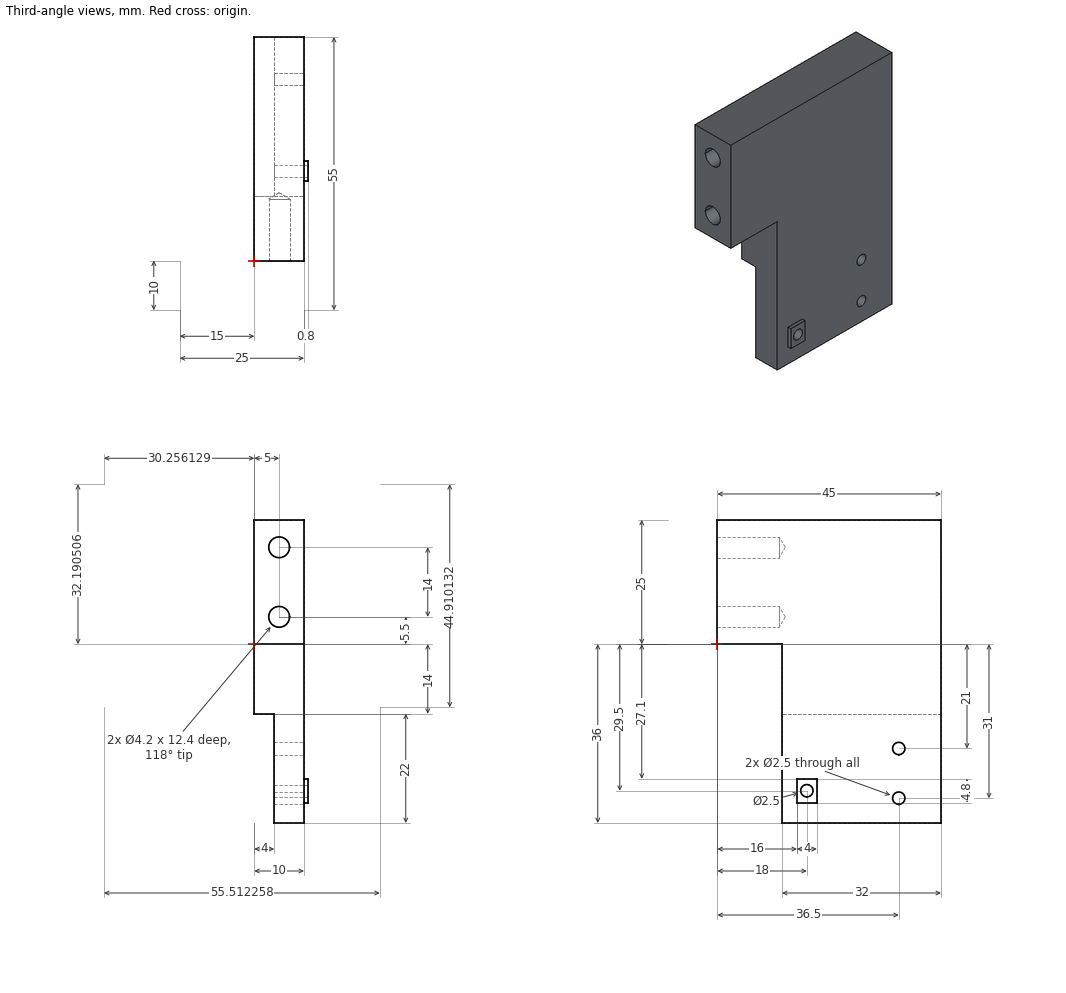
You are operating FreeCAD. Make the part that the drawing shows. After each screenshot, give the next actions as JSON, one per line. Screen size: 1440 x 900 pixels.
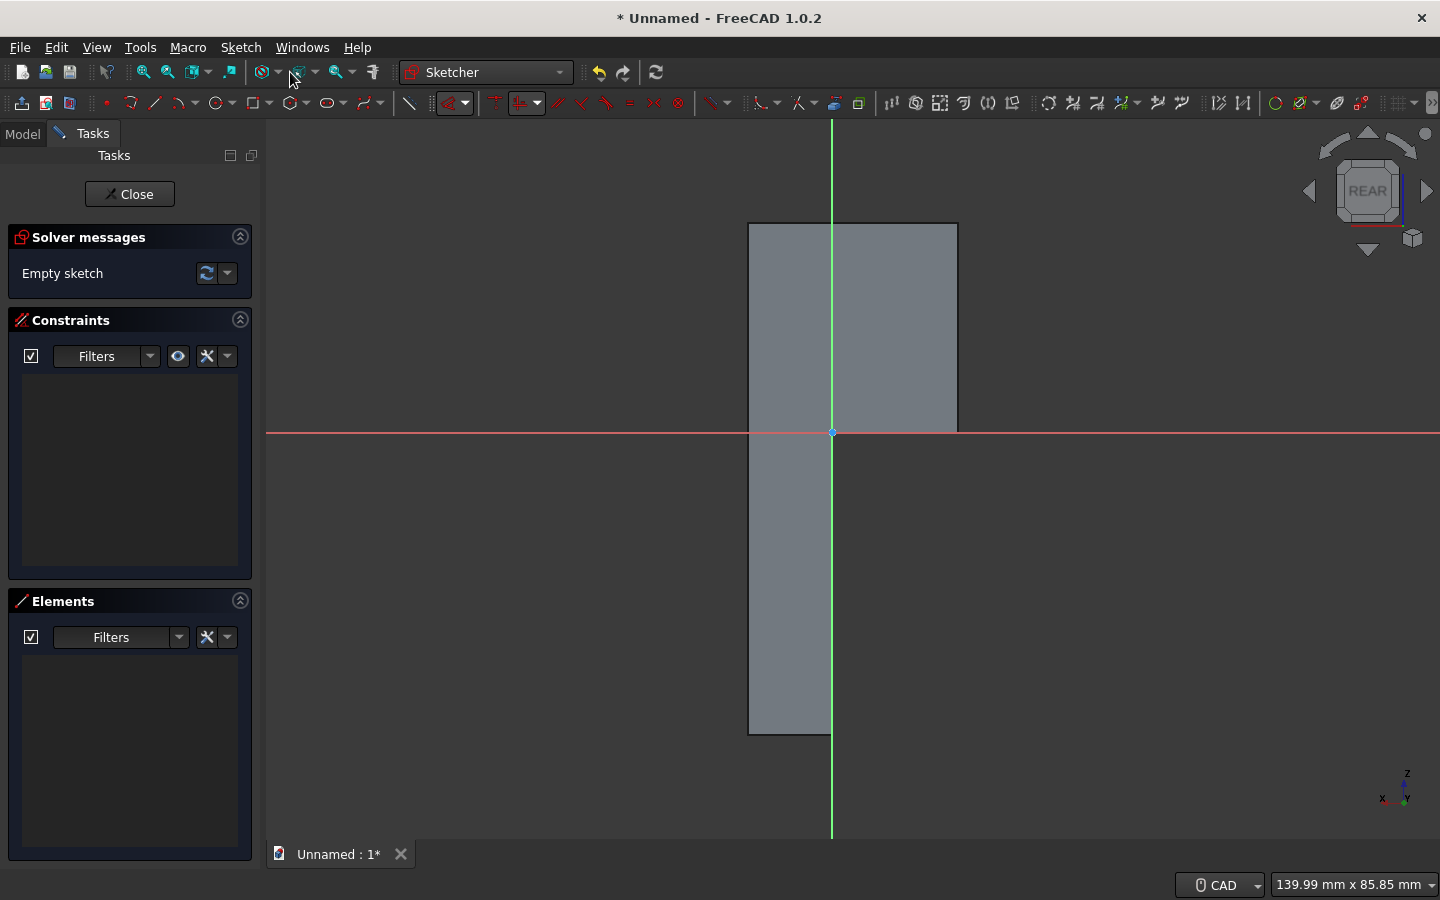
{"action": "scroll", "coordinate": [878, 797], "scroll_direction": "up", "scroll_amount": 2}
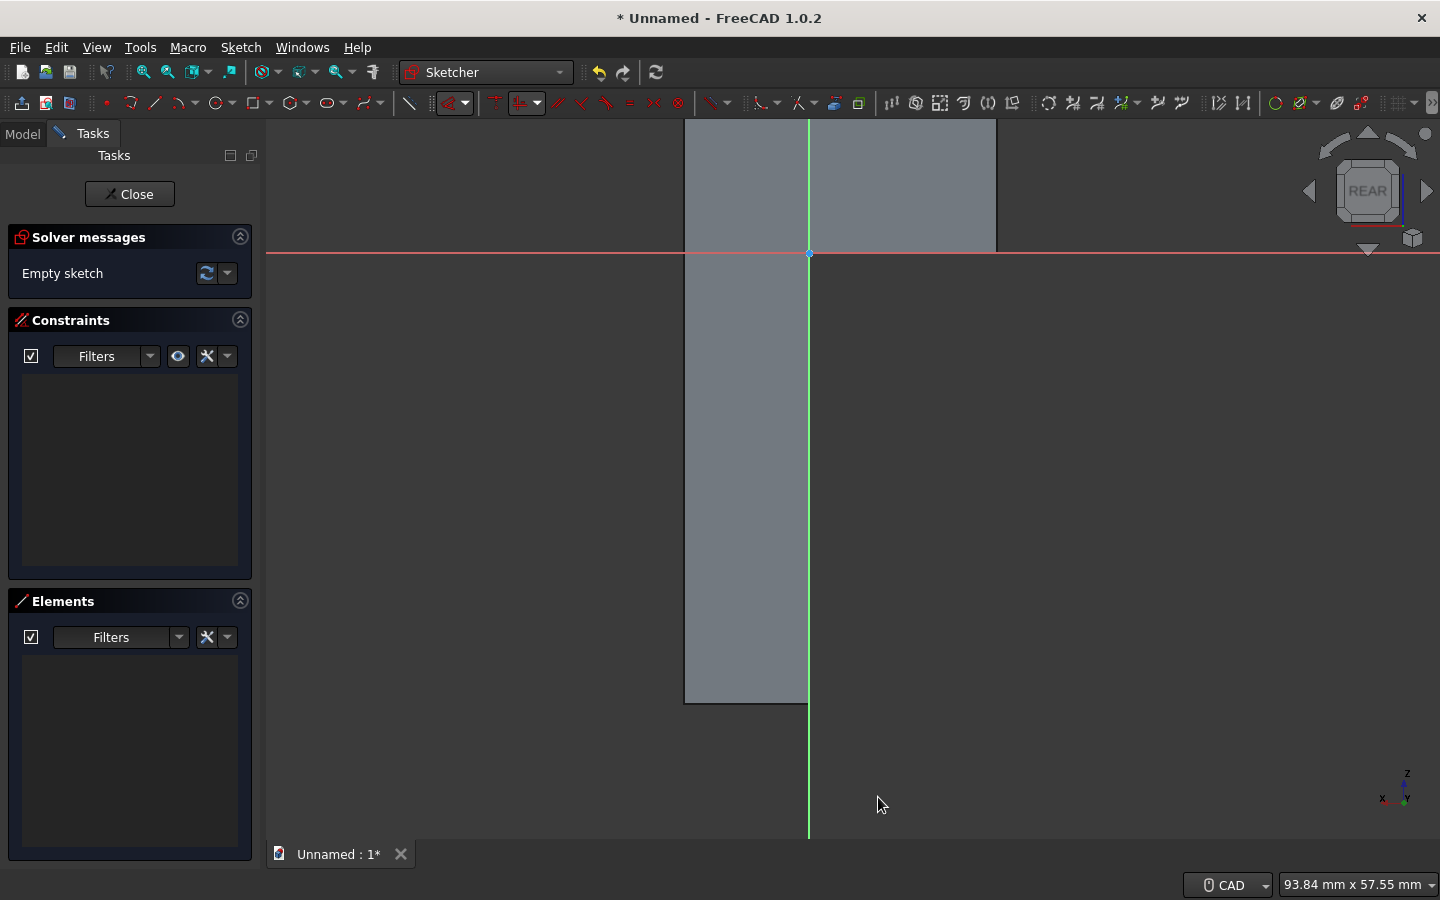
{"action": "key", "text": "g r"}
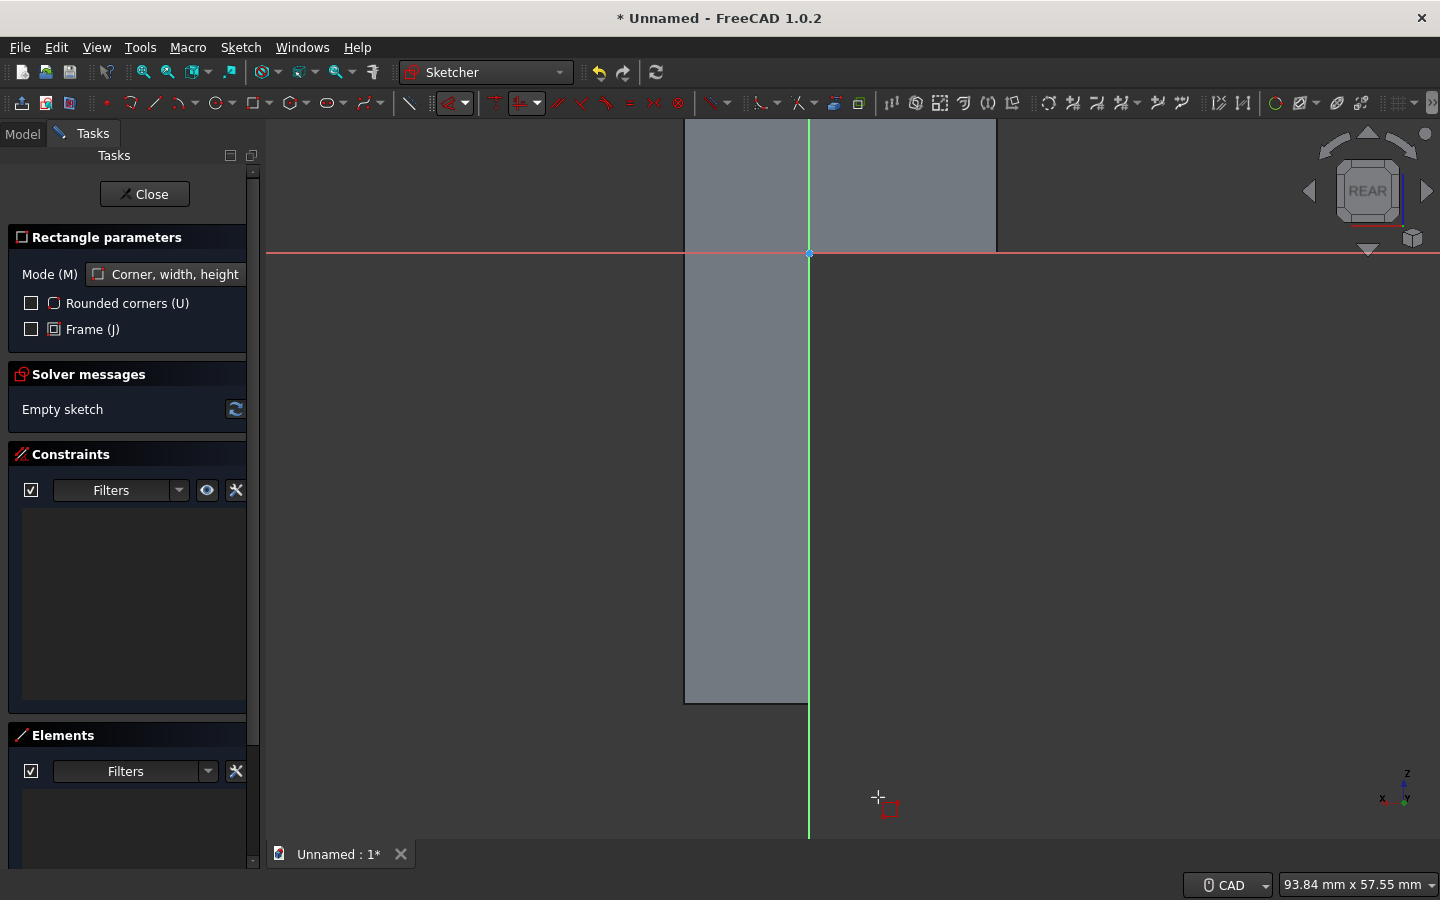
{"action": "left_click", "coordinate": [759, 428]}
{"action": "left_click", "coordinate": [809, 704]}
{"action": "key", "text": "Escape"}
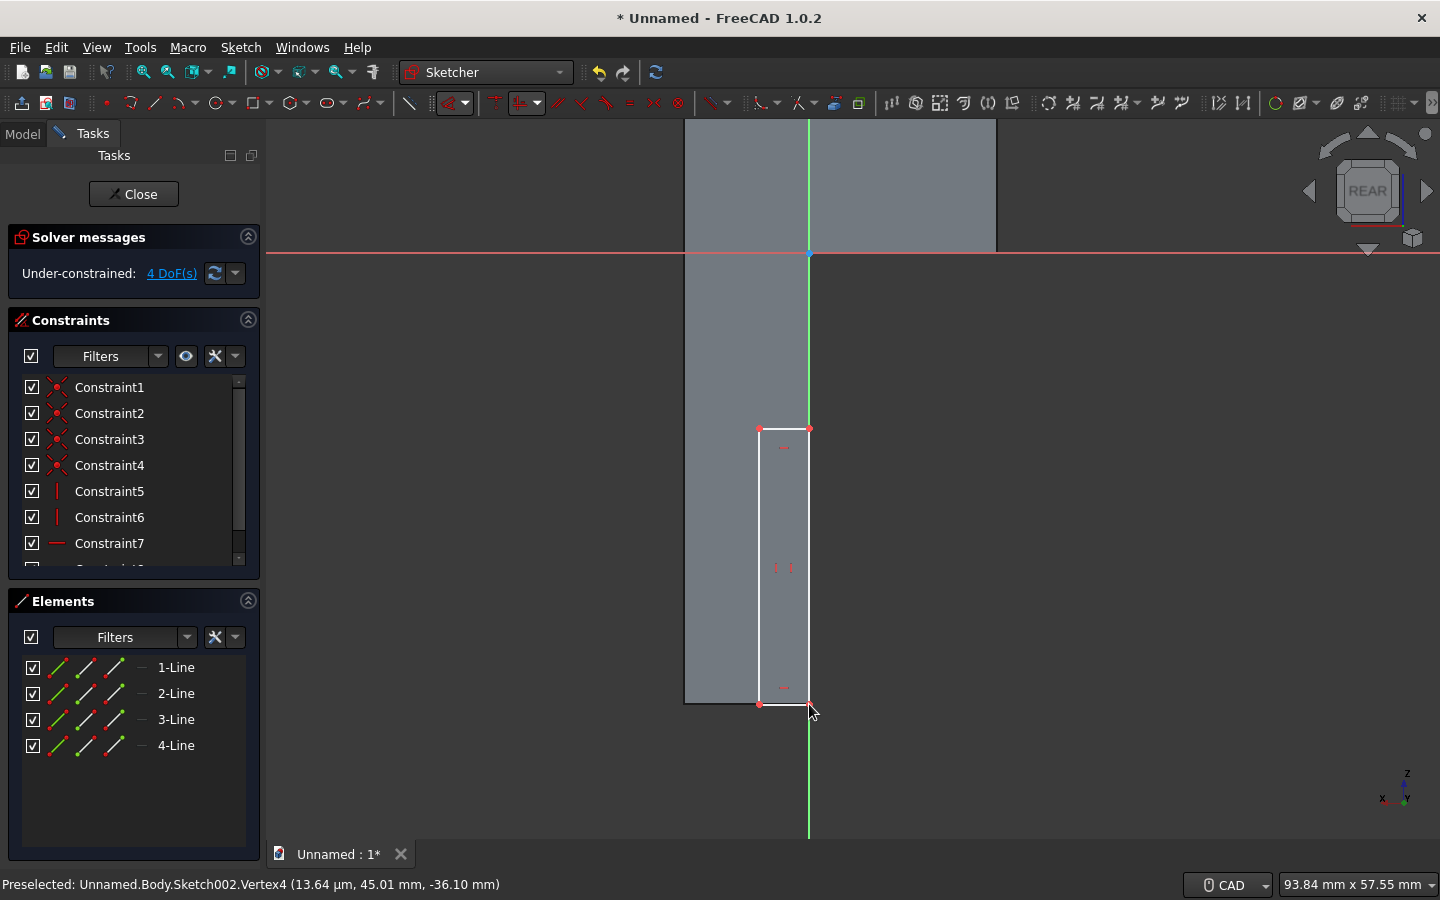
{"action": "left_click", "coordinate": [809, 705]}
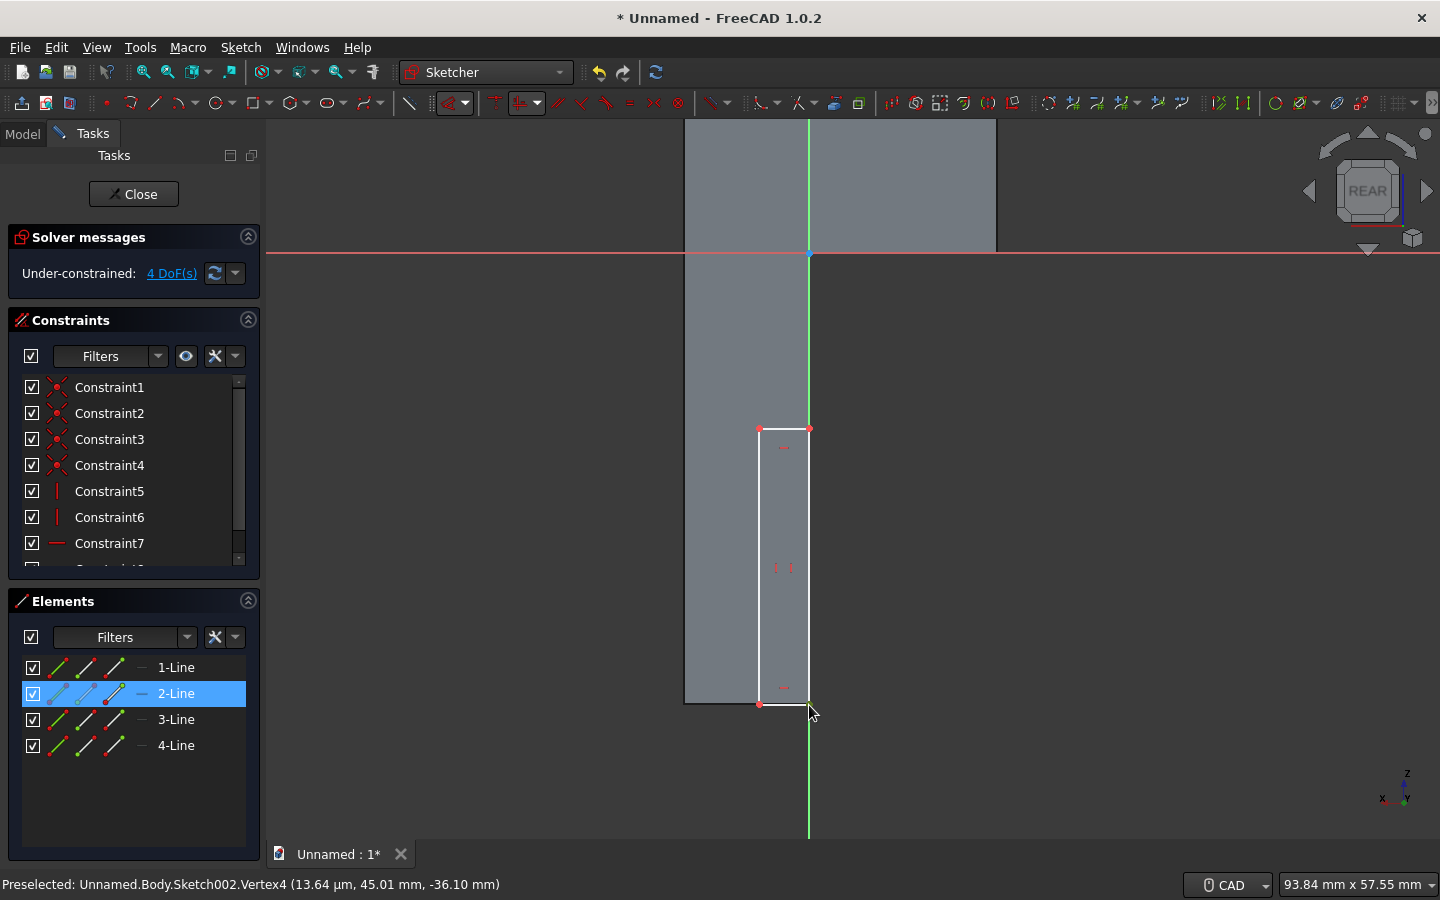
{"action": "left_click", "coordinate": [809, 764]}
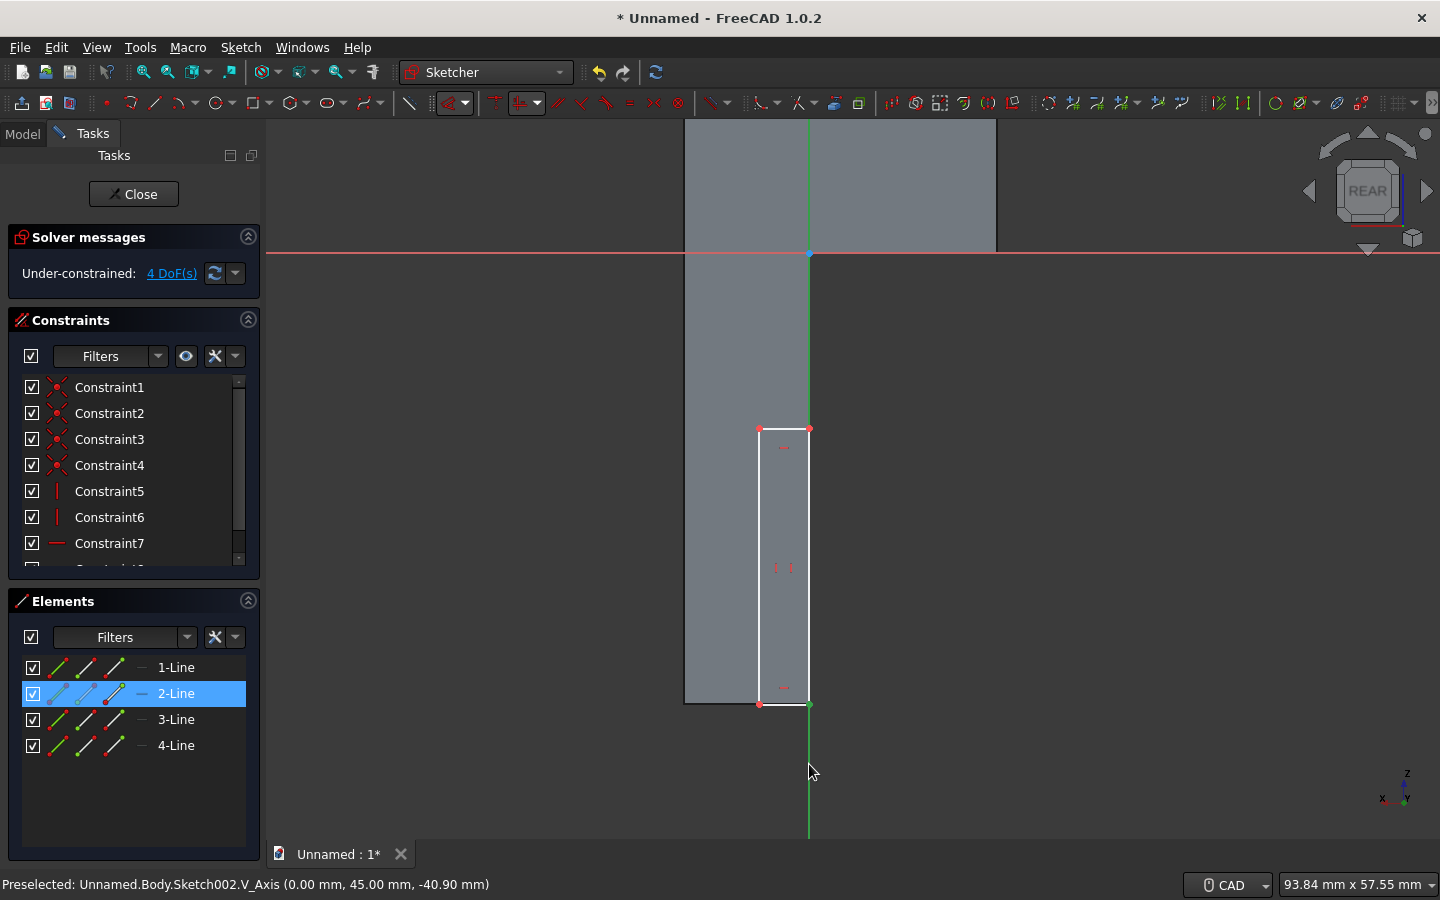
{"action": "key", "text": "c"}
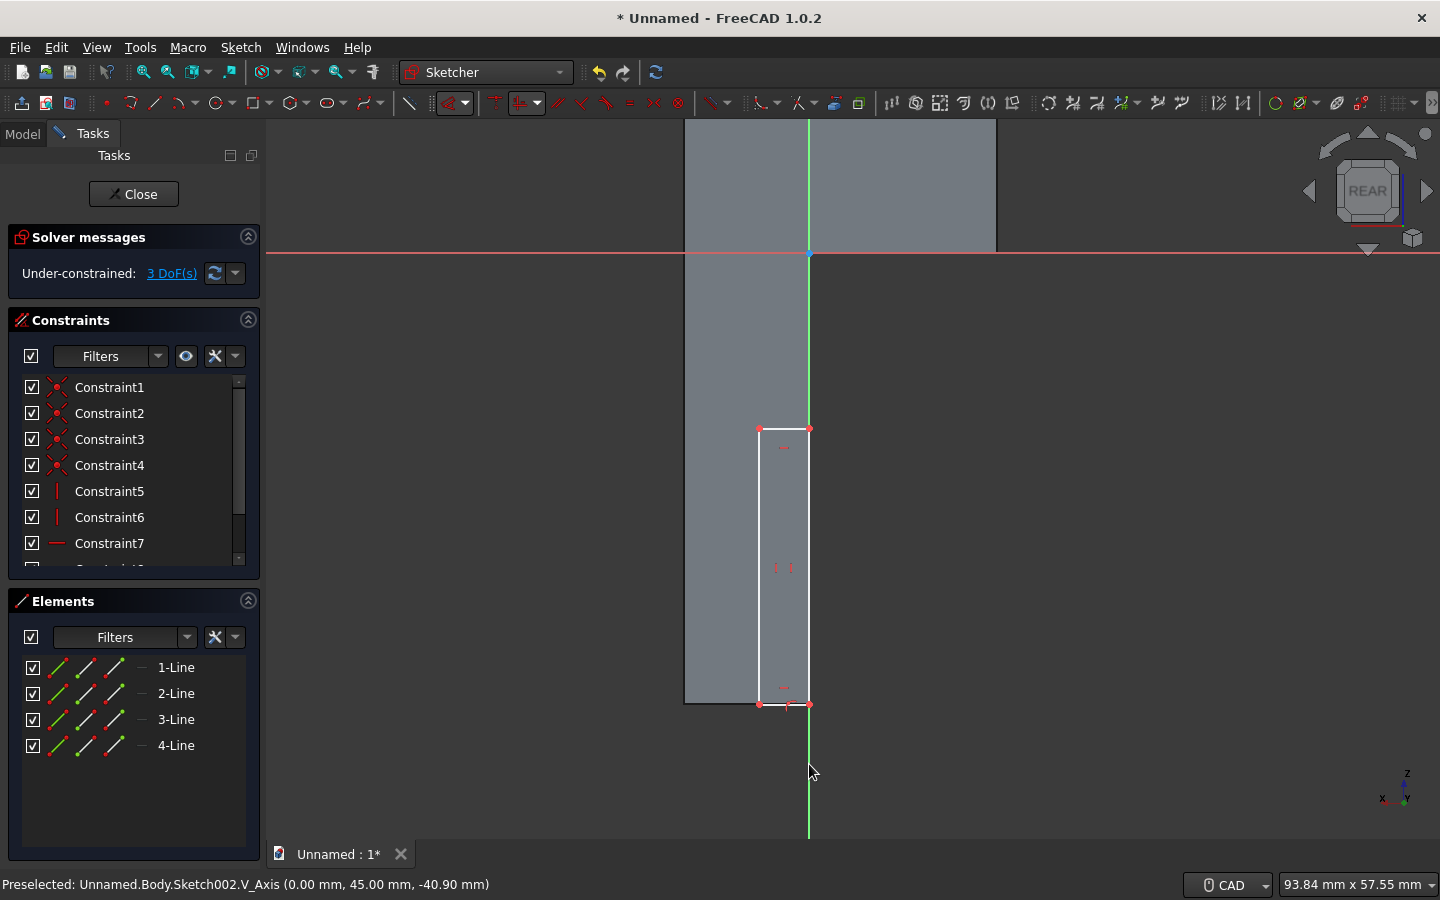
{"action": "left_click", "coordinate": [774, 705]}